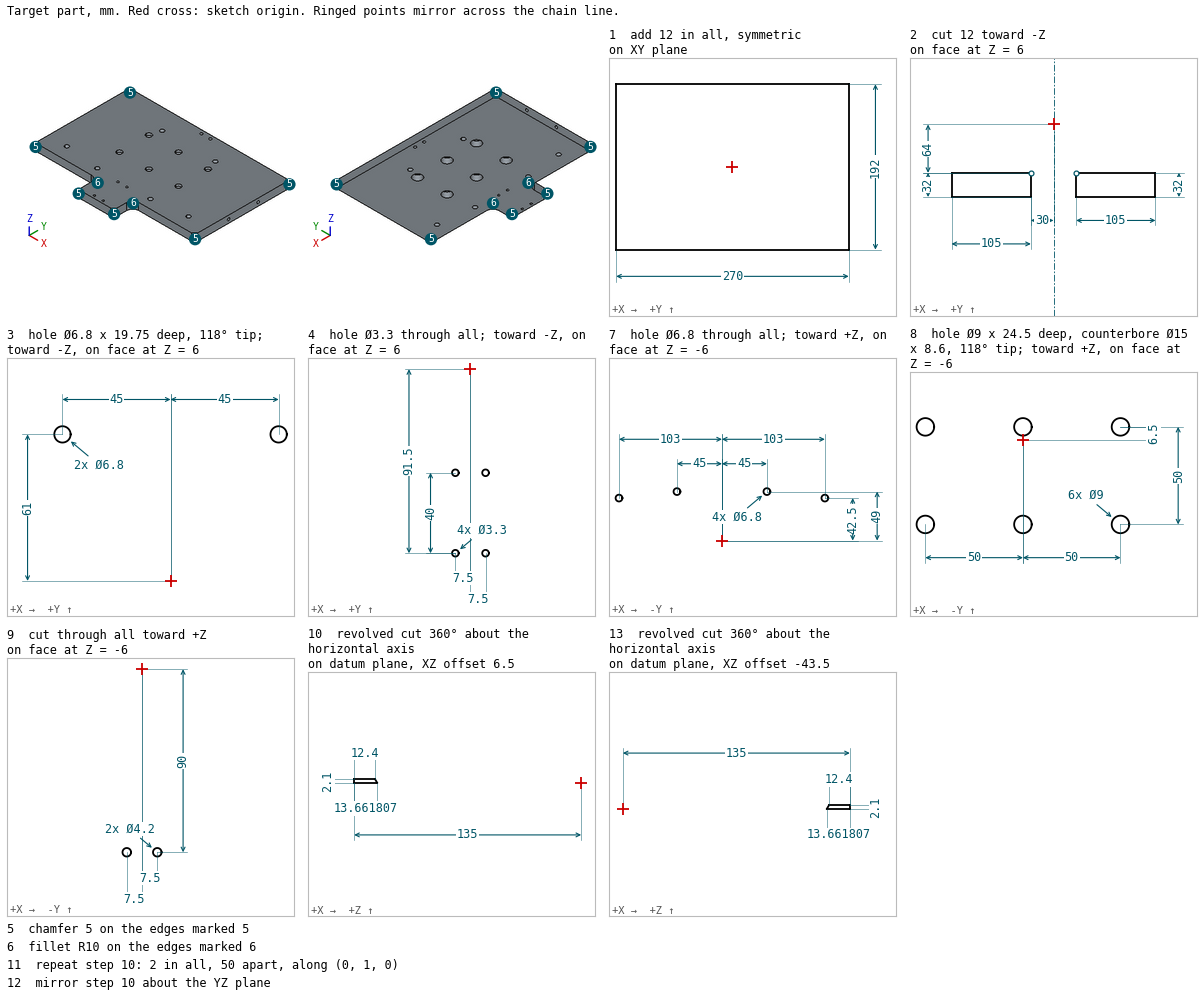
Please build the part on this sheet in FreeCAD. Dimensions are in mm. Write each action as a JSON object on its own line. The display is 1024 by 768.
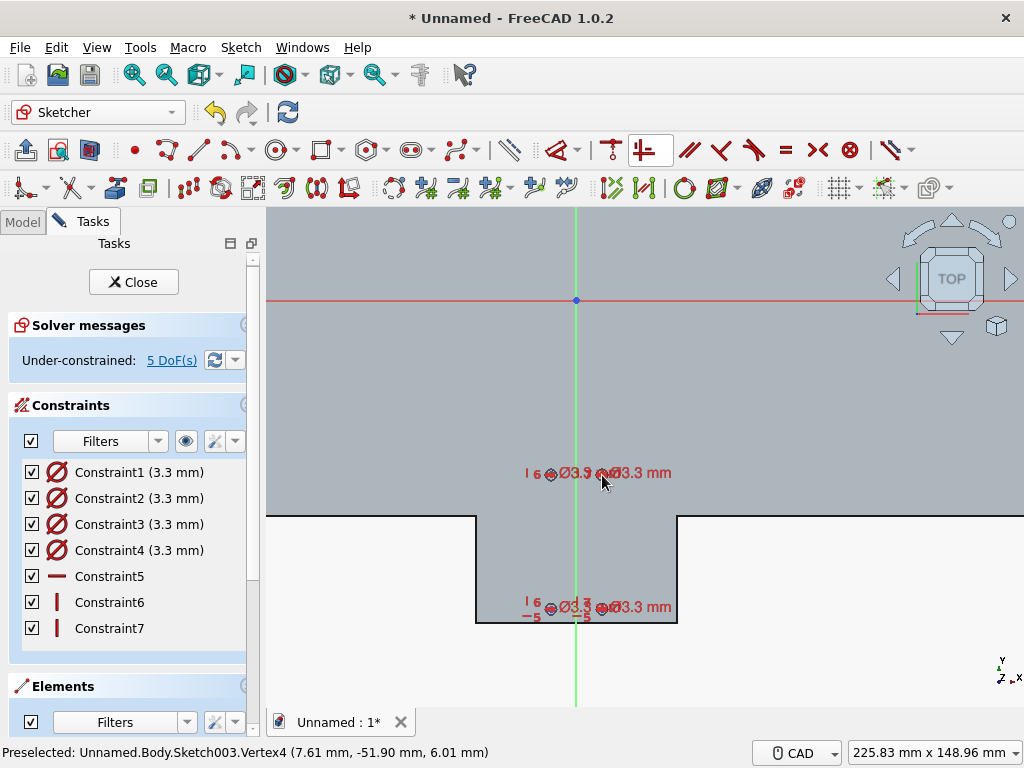
{"action": "key", "text": "h"}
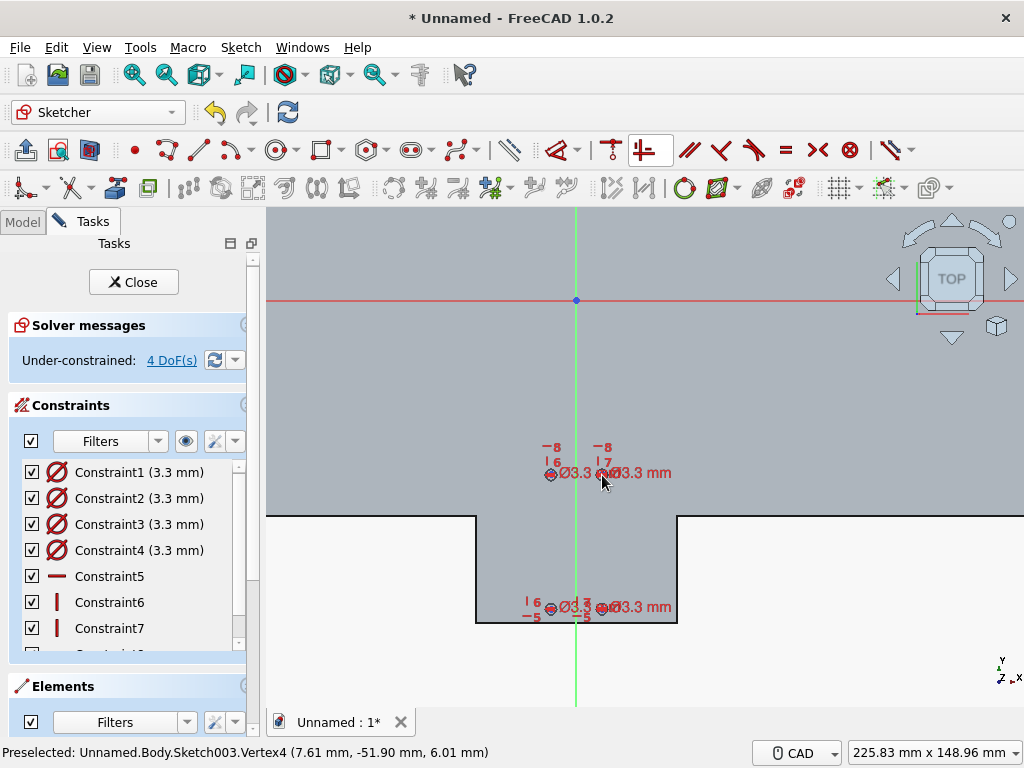
{"action": "left_click", "coordinate": [556, 150]}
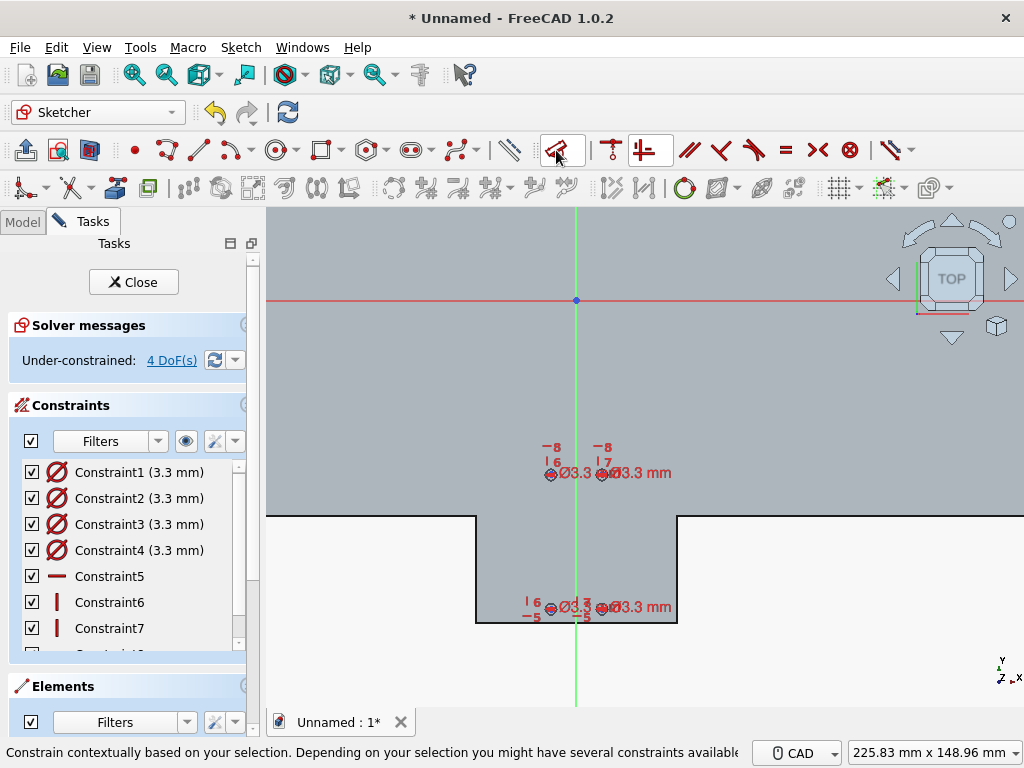
{"action": "scroll", "coordinate": [551, 609], "scroll_direction": "up", "scroll_amount": 3}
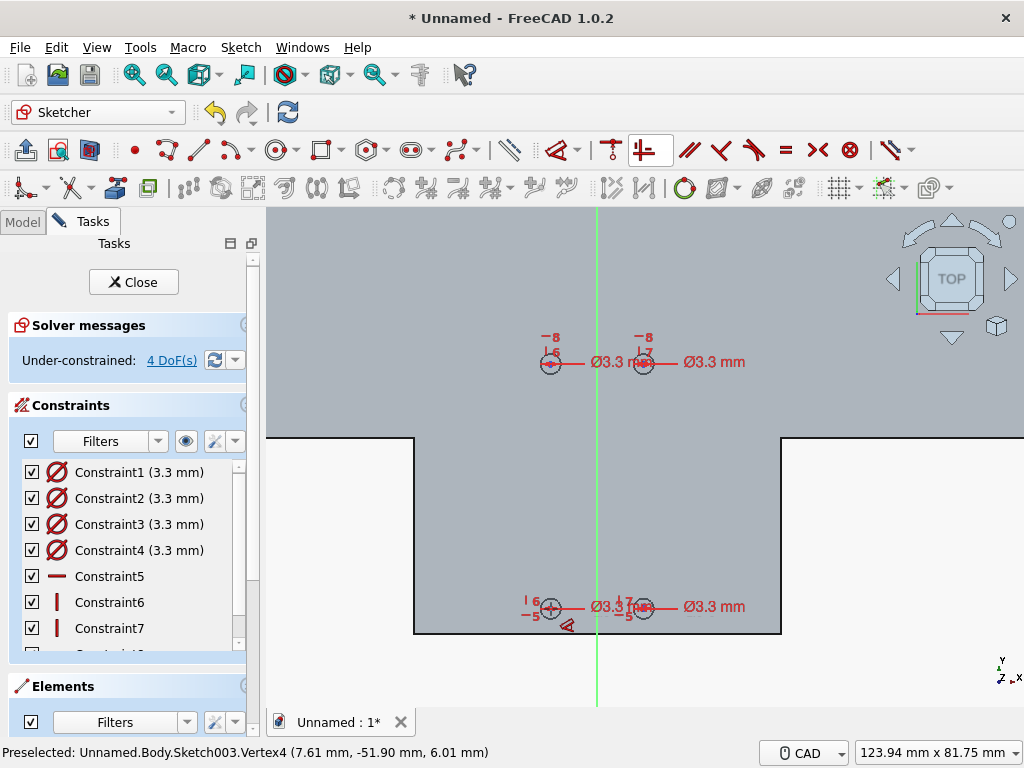
{"action": "left_click", "coordinate": [551, 609]}
{"action": "left_click", "coordinate": [574, 643]}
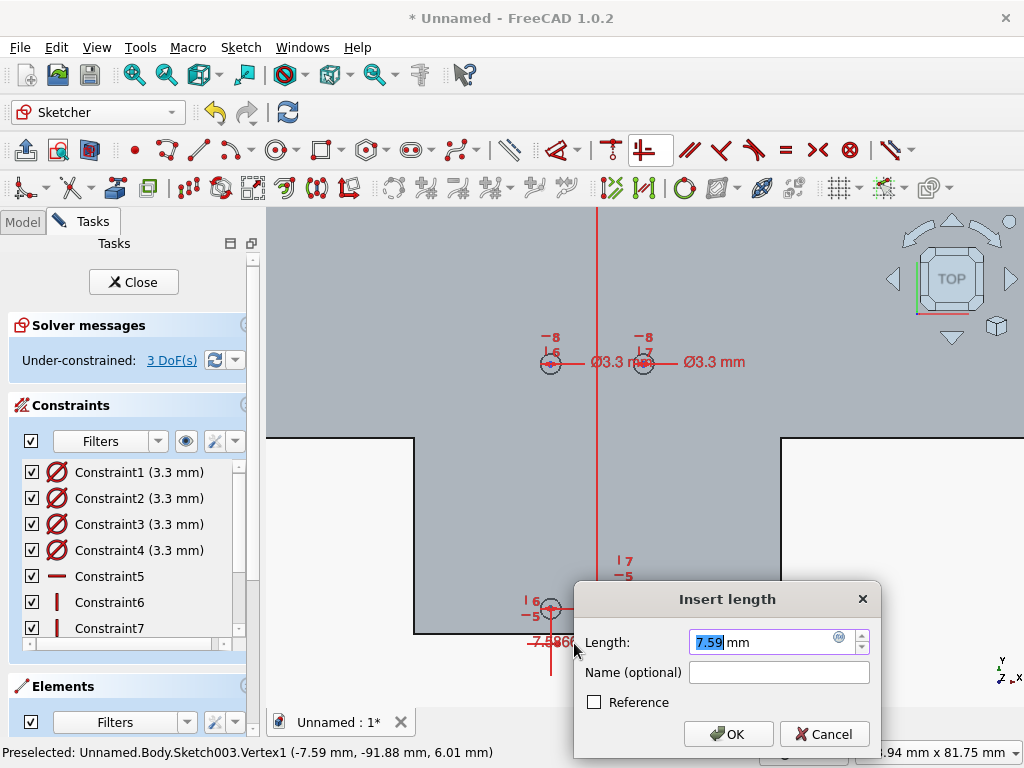
{"action": "type", "text": "7.5"}
{"action": "key", "text": "Return"}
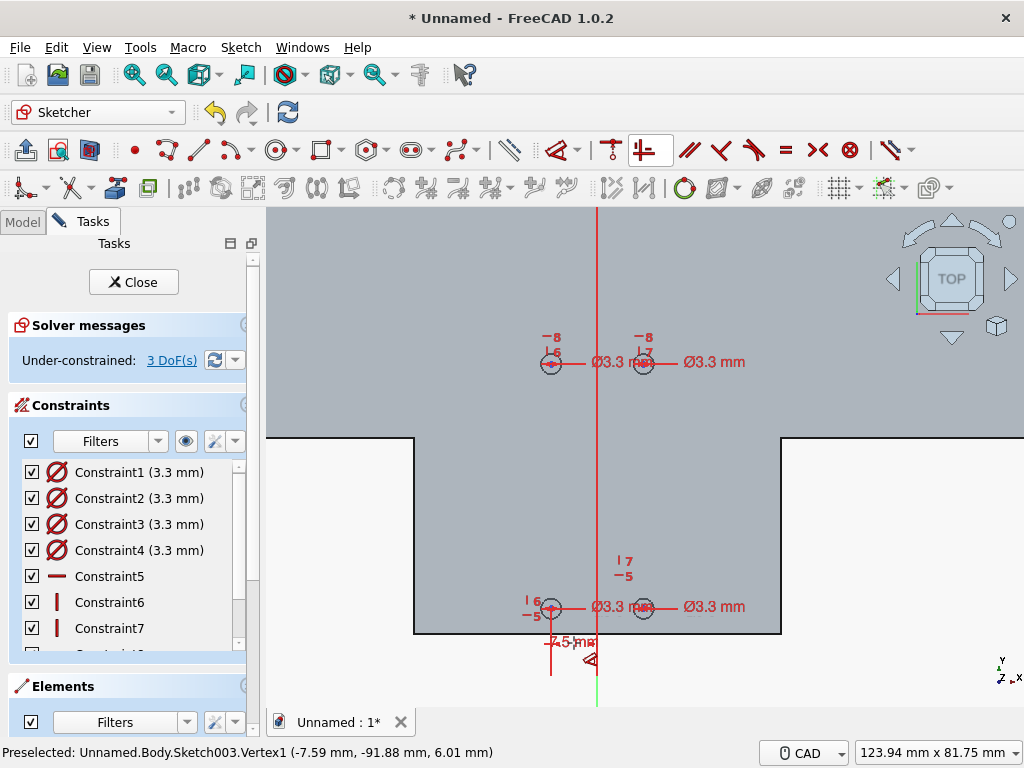
{"action": "left_click", "coordinate": [644, 609]}
{"action": "left_click", "coordinate": [620, 667]}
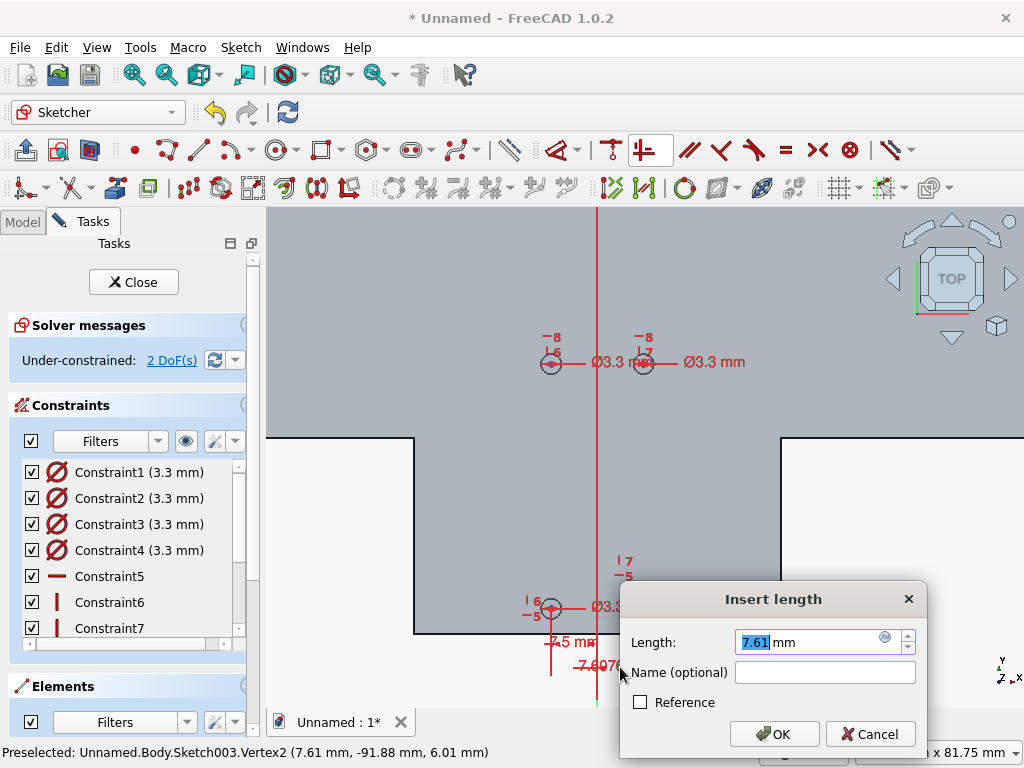
{"action": "type", "text": "7.5"}
{"action": "key", "text": "Return"}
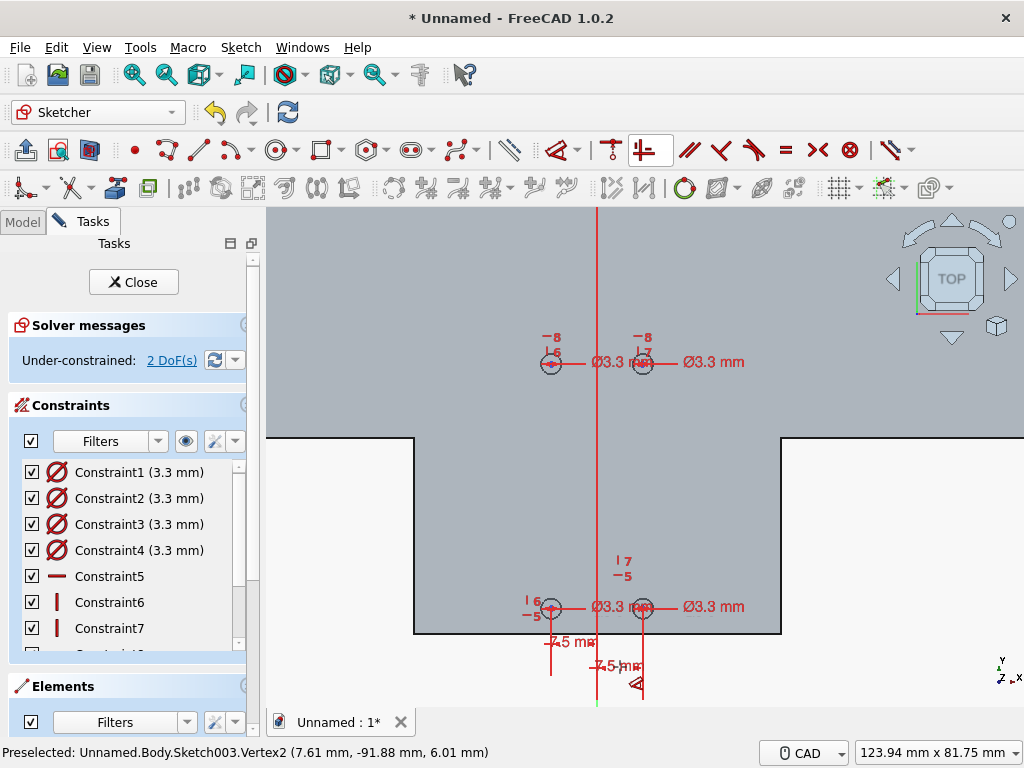
{"action": "left_click", "coordinate": [551, 609]}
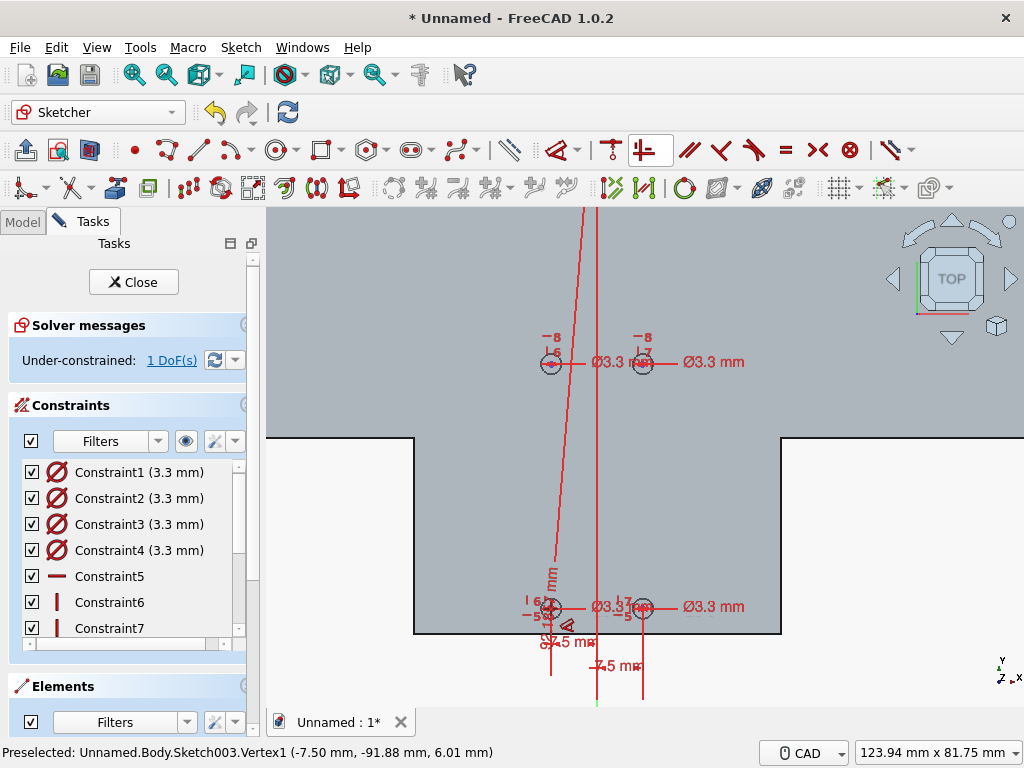
{"action": "left_click", "coordinate": [551, 364]}
{"action": "left_click", "coordinate": [517, 486]}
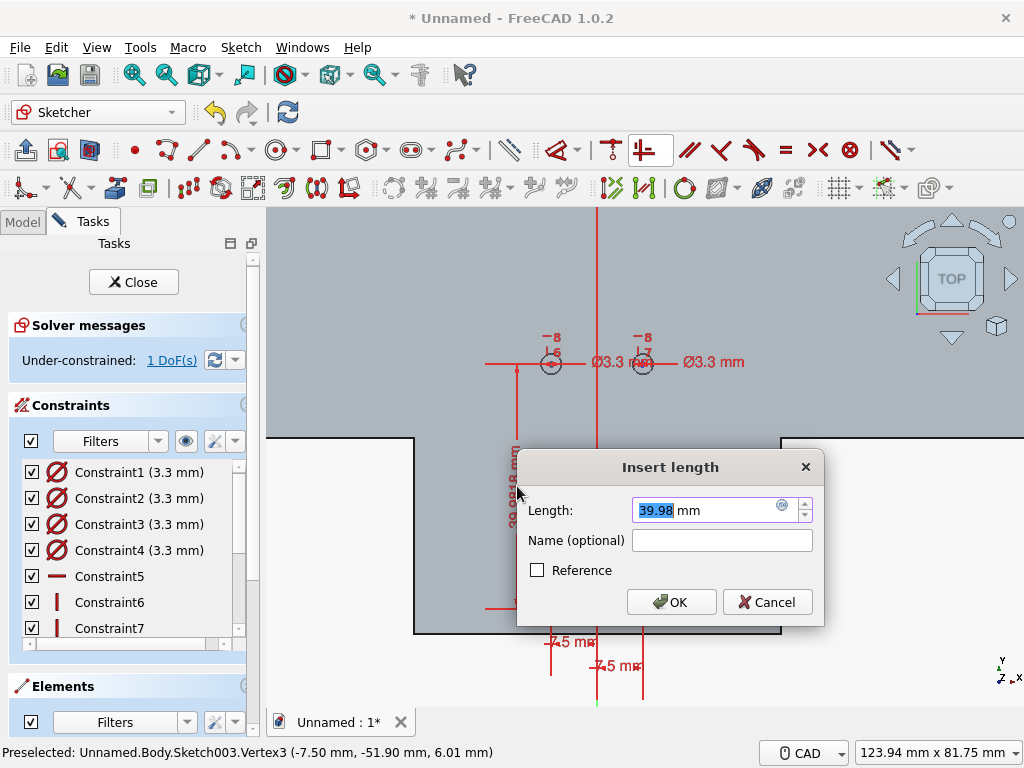
{"action": "type", "text": "40"}
{"action": "key", "text": "Return"}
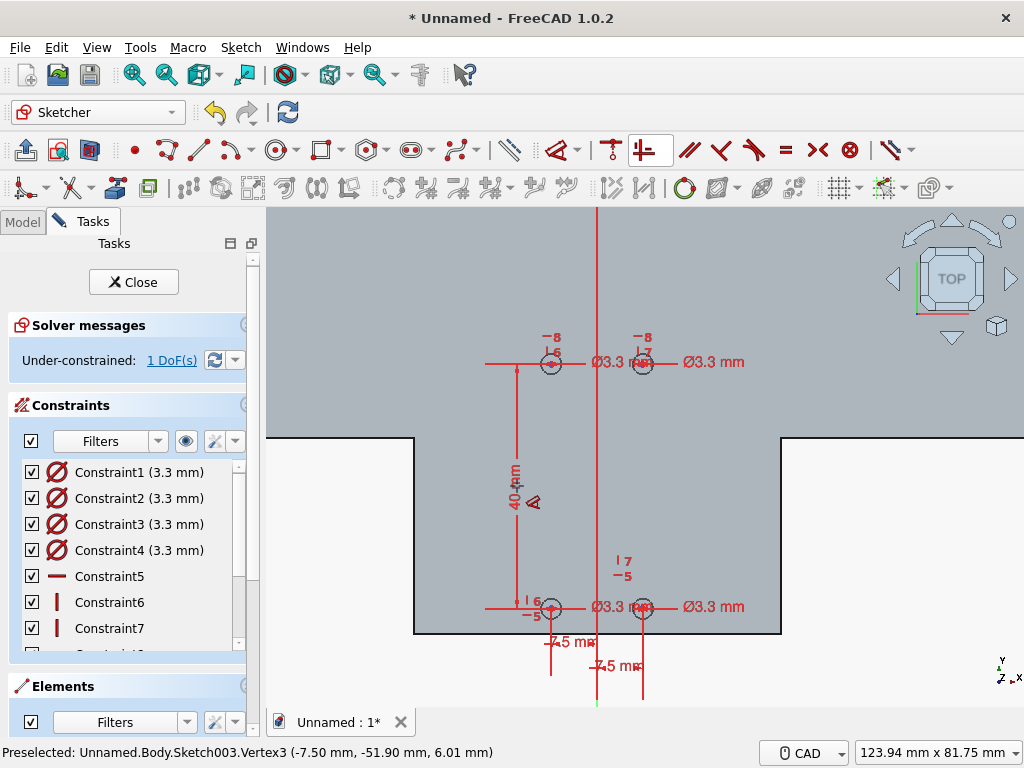
{"action": "left_click", "coordinate": [551, 609]}
{"action": "left_click", "coordinate": [517, 422]}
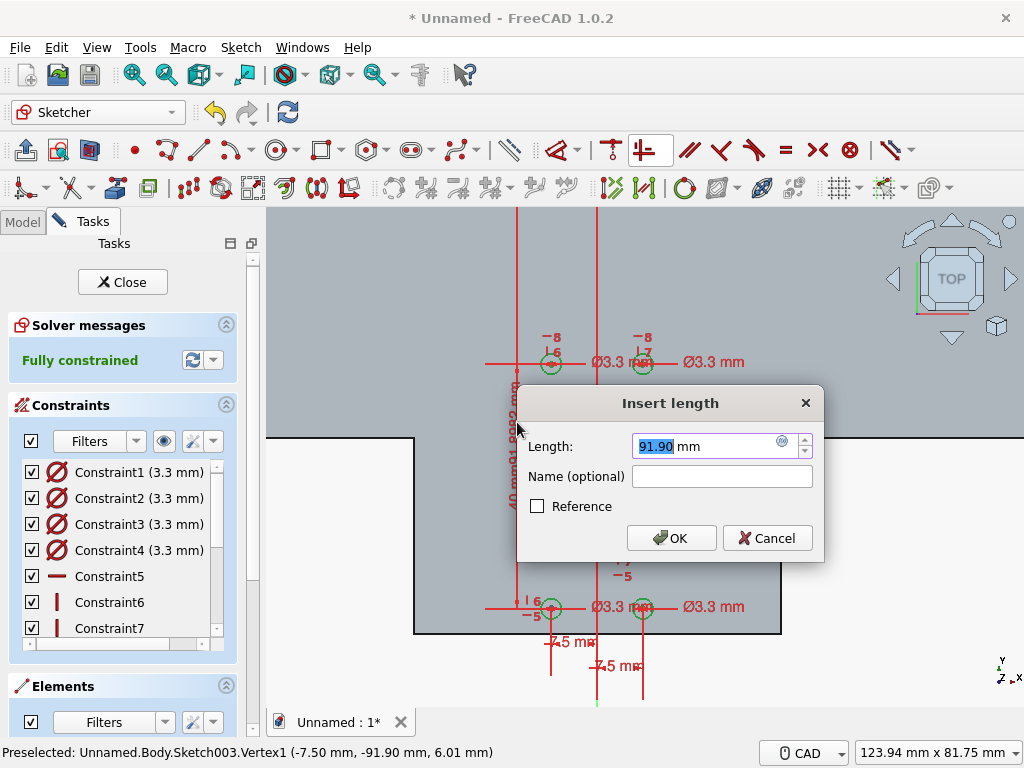
{"action": "type", "text": "91.5"}
{"action": "key", "text": "Return"}
{"action": "key", "text": "Escape"}